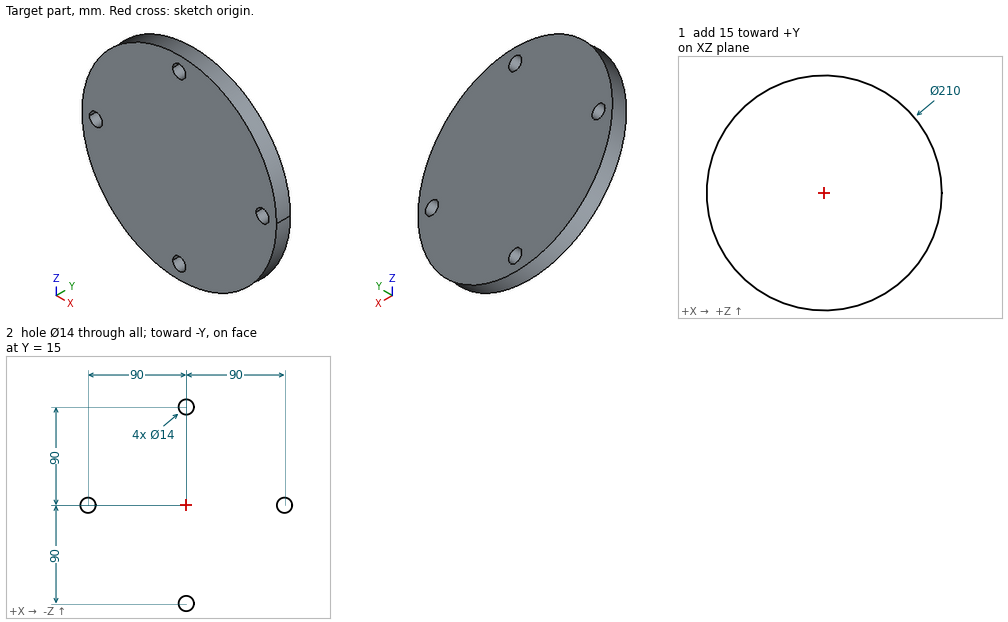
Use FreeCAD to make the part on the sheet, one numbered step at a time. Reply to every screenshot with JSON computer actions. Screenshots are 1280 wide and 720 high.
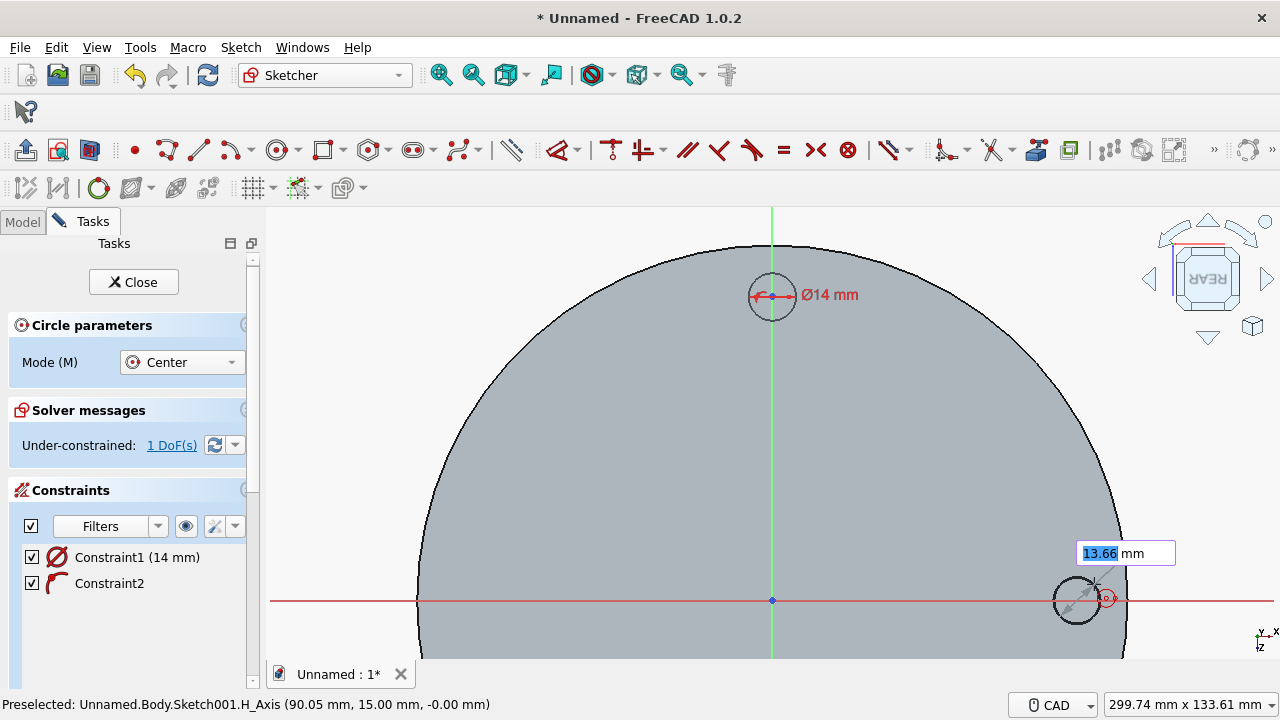
{"action": "type", "text": "14"}
{"action": "key", "text": "Return"}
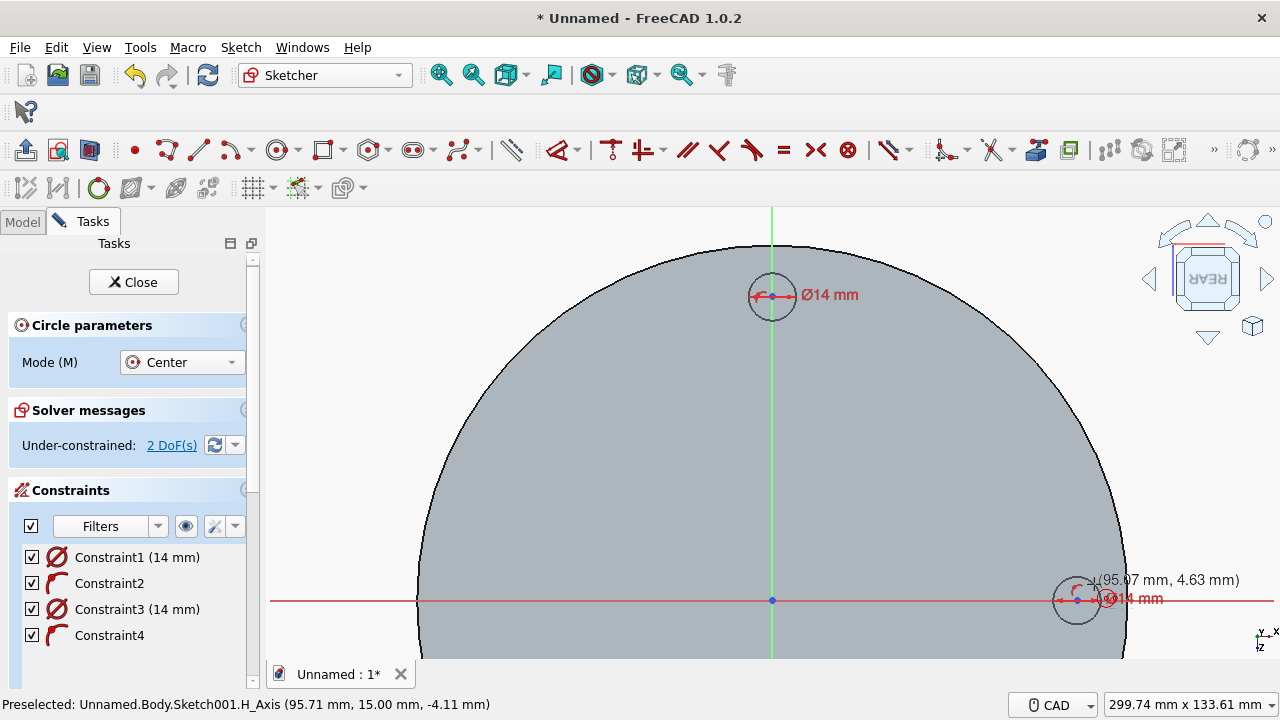
{"action": "scroll", "coordinate": [649, 296], "scroll_direction": "down", "scroll_amount": 4}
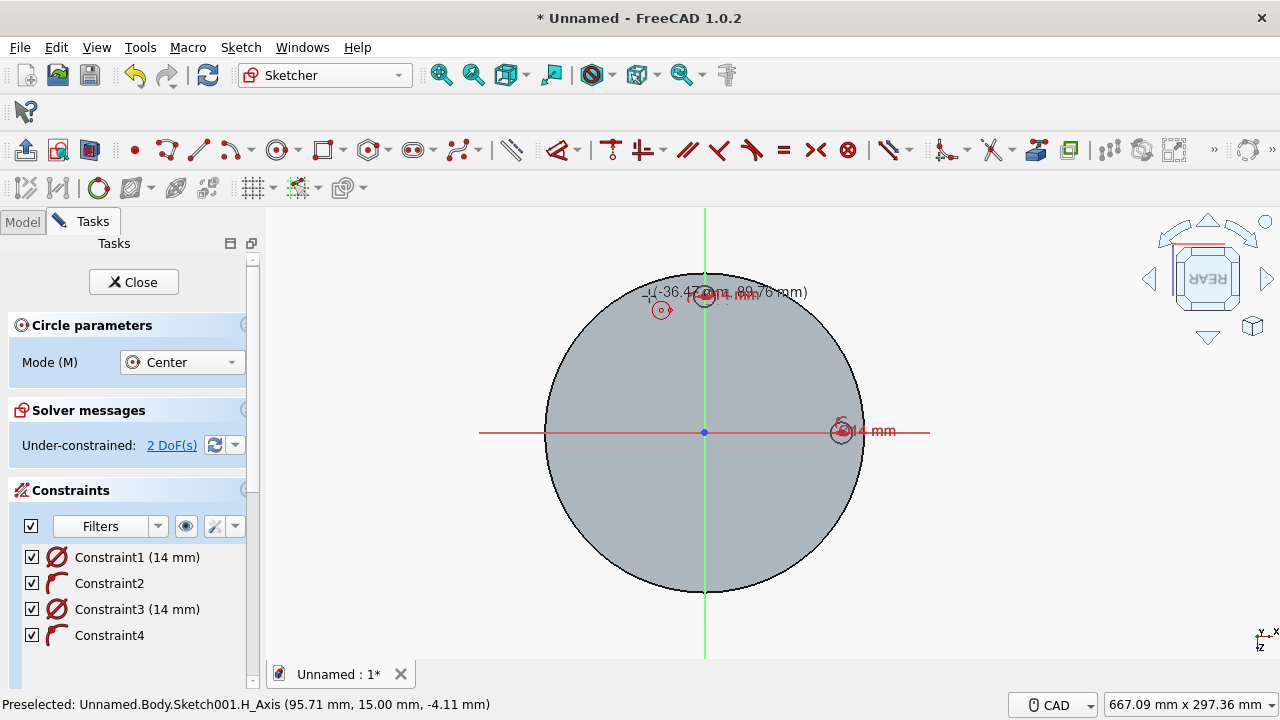
{"action": "scroll", "coordinate": [705, 570], "scroll_direction": "up", "scroll_amount": 4}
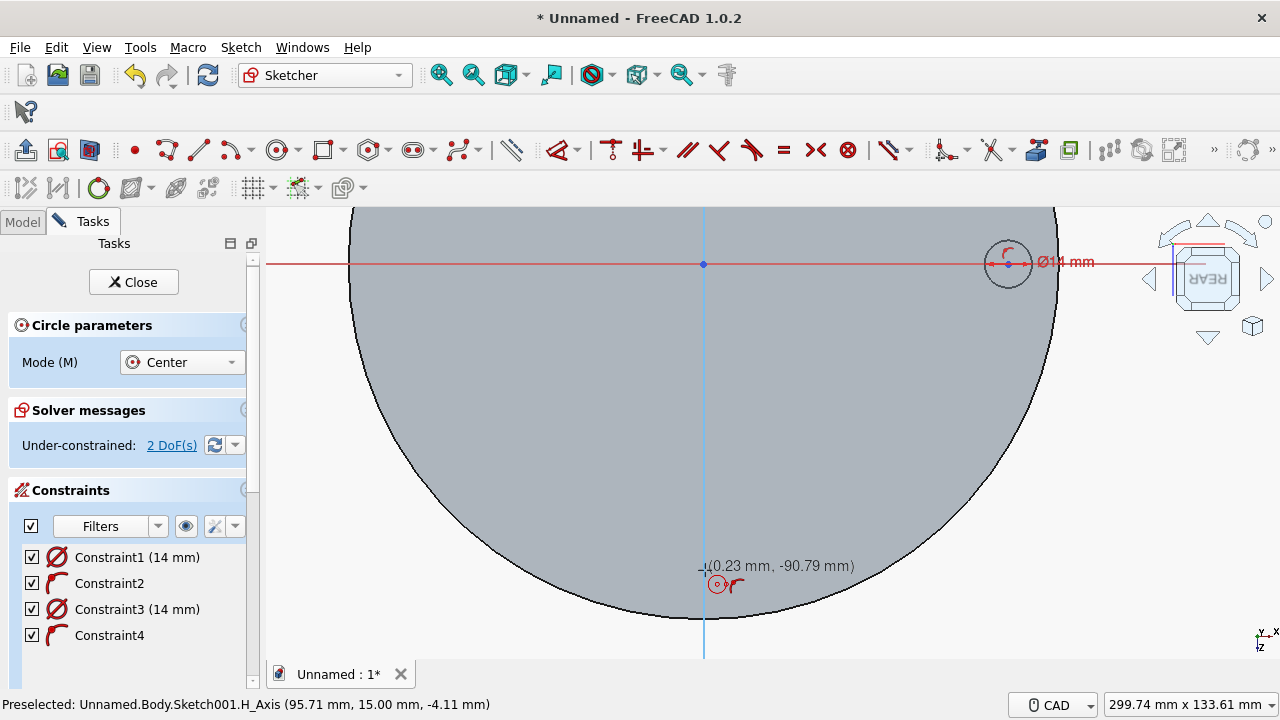
{"action": "left_click", "coordinate": [704, 569]}
{"action": "mouse_move", "coordinate": [720, 552]}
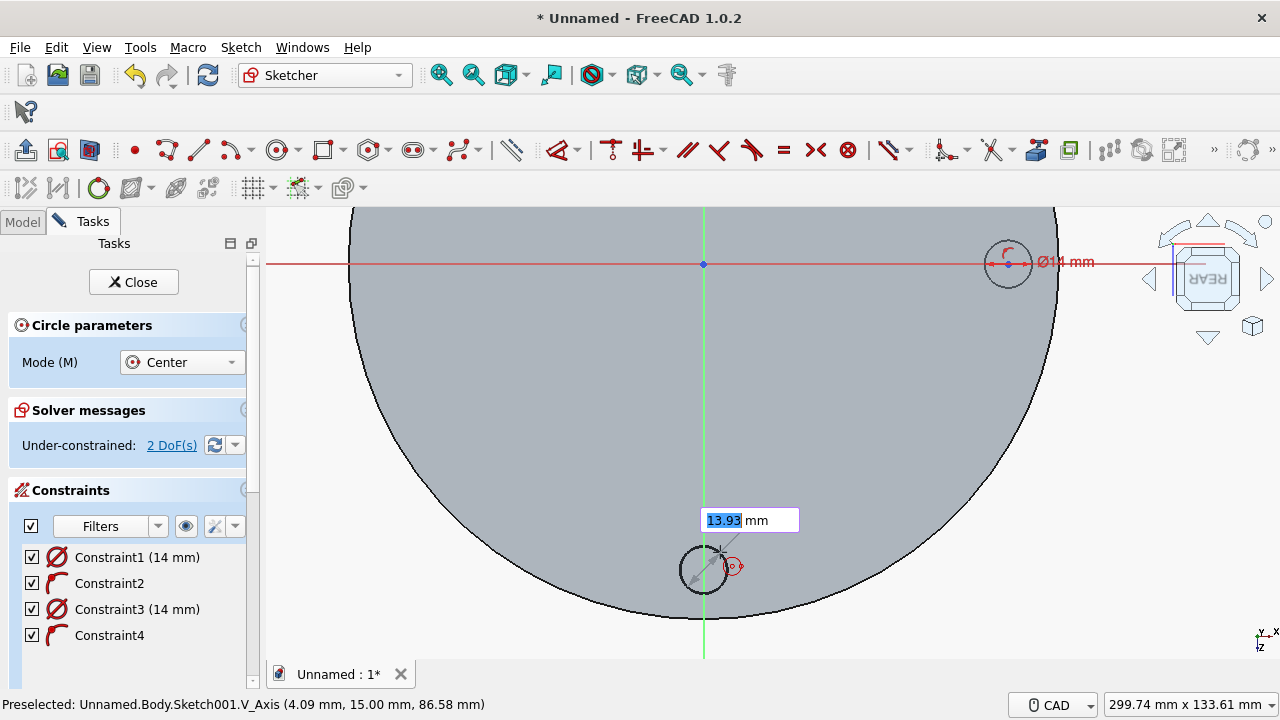
{"action": "type", "text": "14"}
{"action": "key", "text": "Return"}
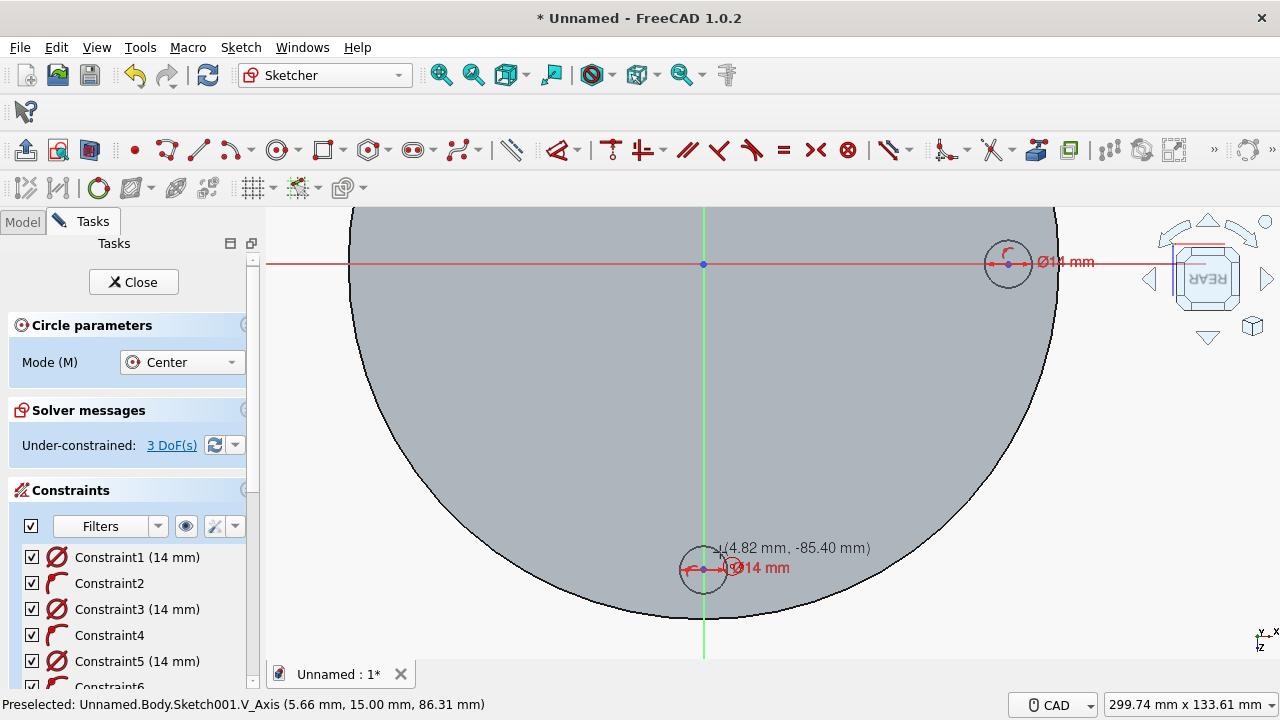
{"action": "left_click", "coordinate": [399, 264]}
{"action": "mouse_move", "coordinate": [416, 247]}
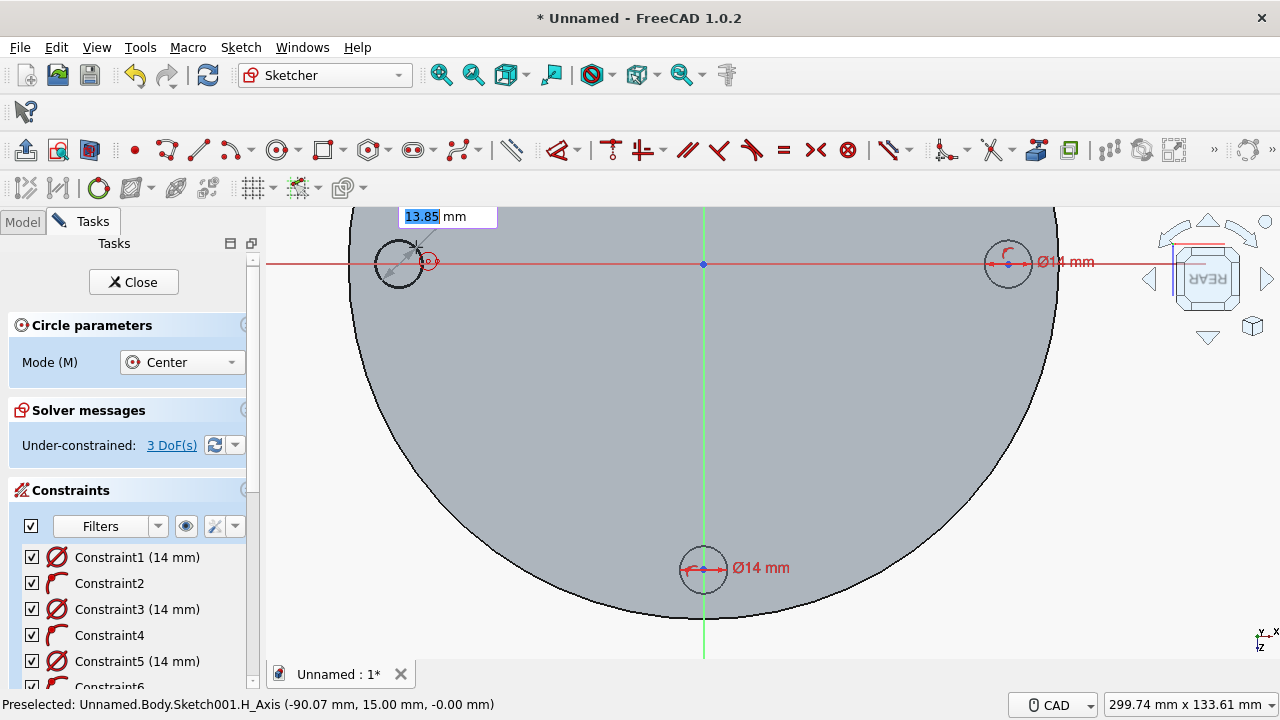
{"action": "type", "text": "14"}
{"action": "key", "text": "Return"}
{"action": "key", "text": "Escape"}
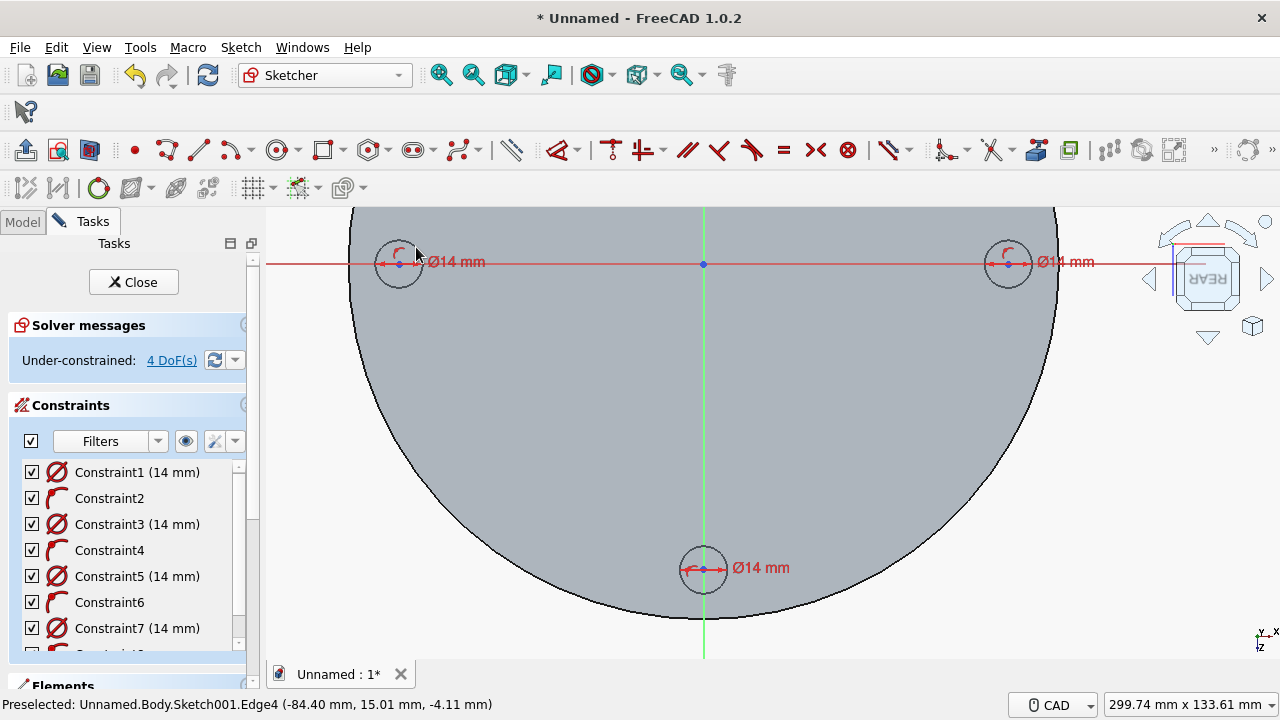
{"action": "left_click", "coordinate": [558, 150]}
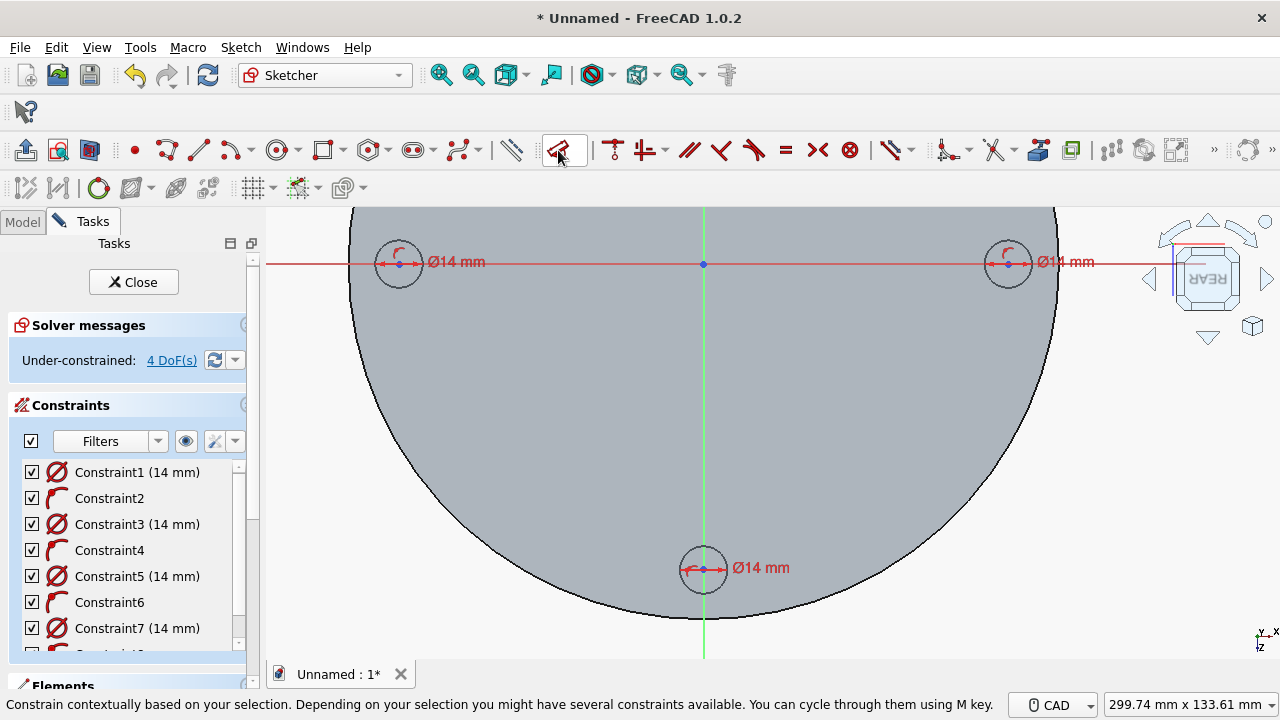
{"action": "scroll", "coordinate": [705, 571], "scroll_direction": "down", "scroll_amount": 4}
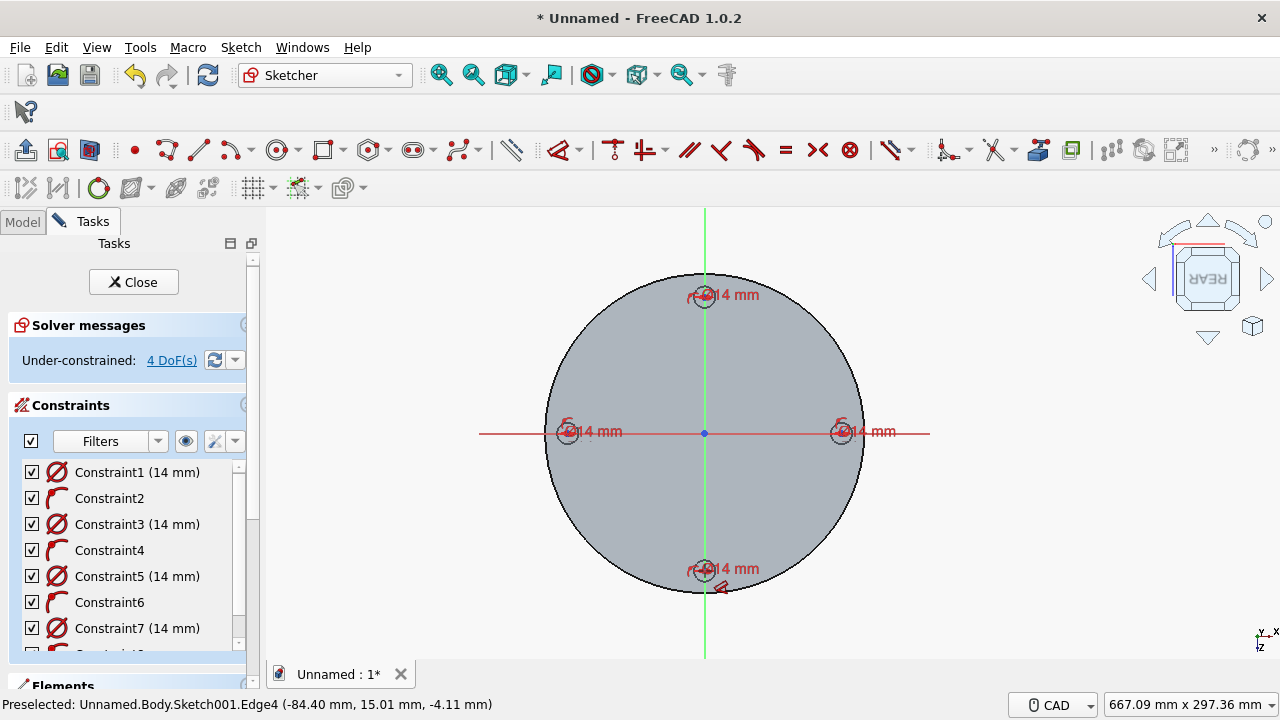
{"action": "left_click", "coordinate": [705, 297]}
{"action": "left_click", "coordinate": [739, 365]}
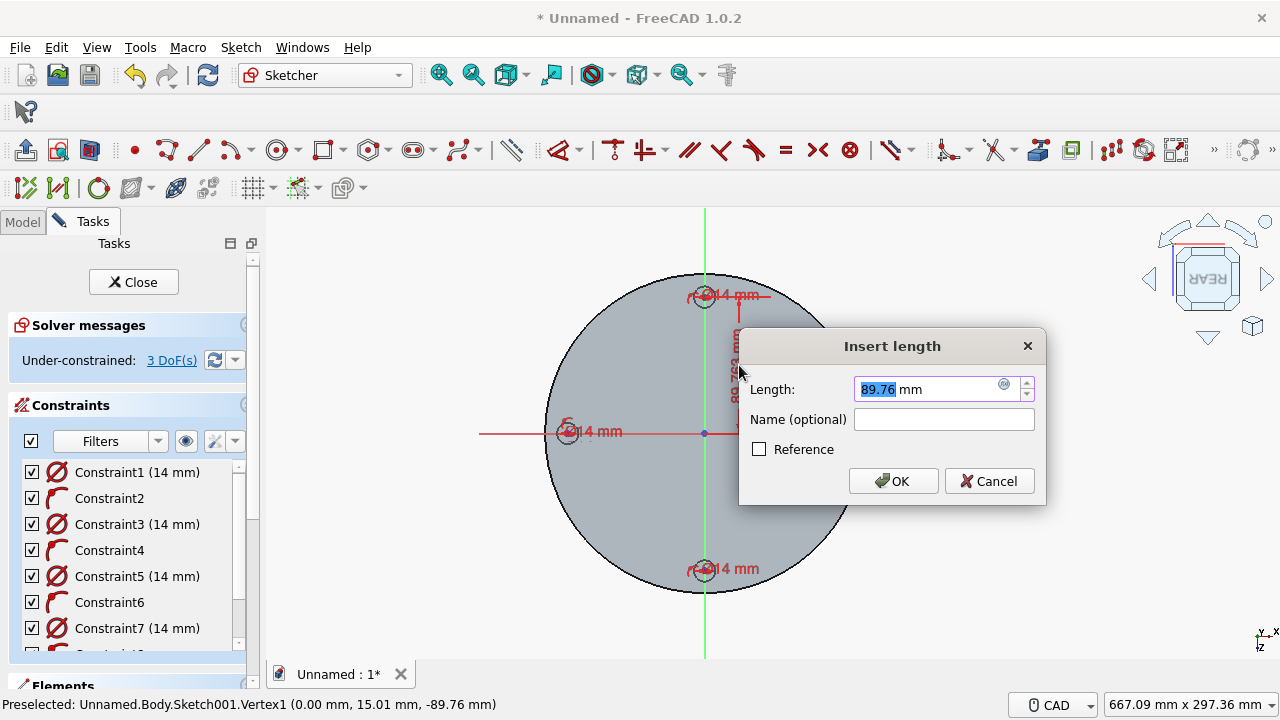
{"action": "type", "text": "90"}
{"action": "key", "text": "Return"}